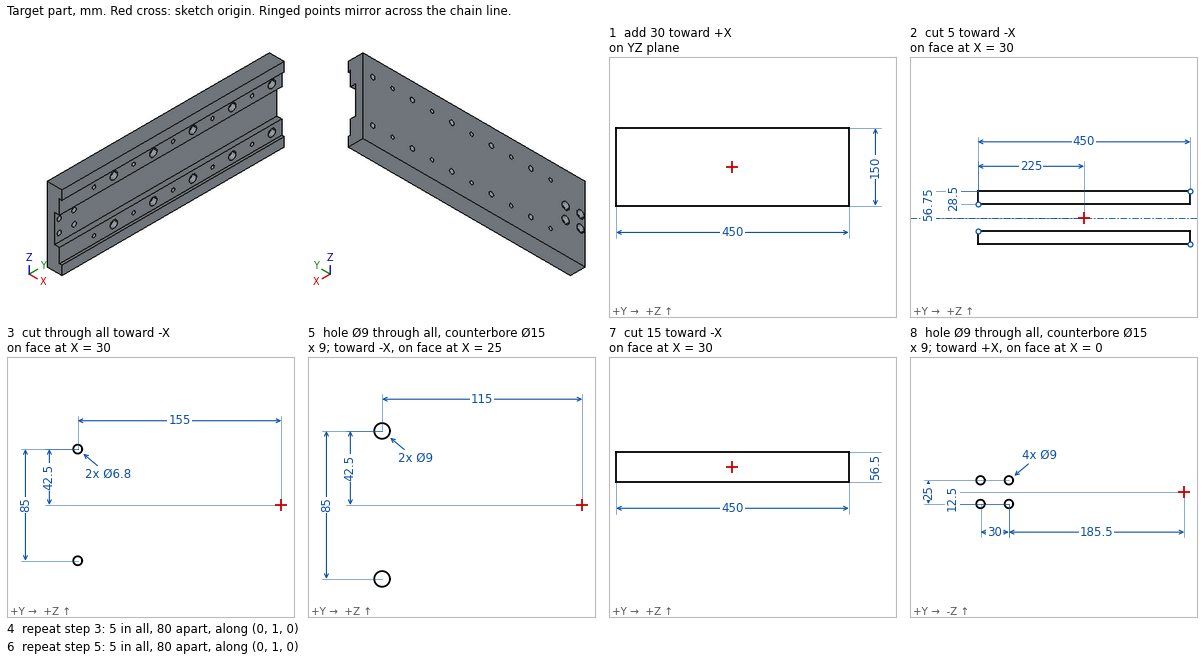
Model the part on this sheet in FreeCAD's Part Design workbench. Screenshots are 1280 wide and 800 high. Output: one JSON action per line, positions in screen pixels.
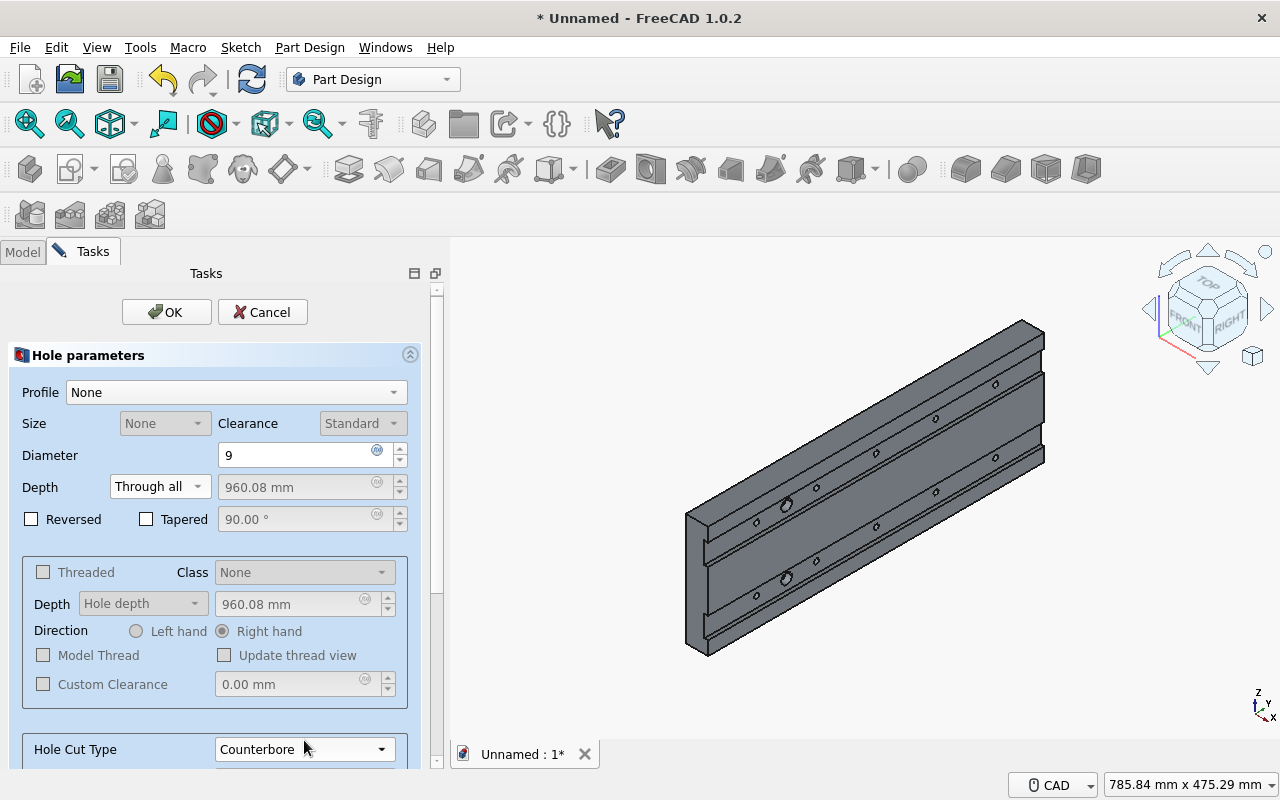
{"action": "scroll", "coordinate": [437, 526], "scroll_direction": "down", "scroll_amount": 2}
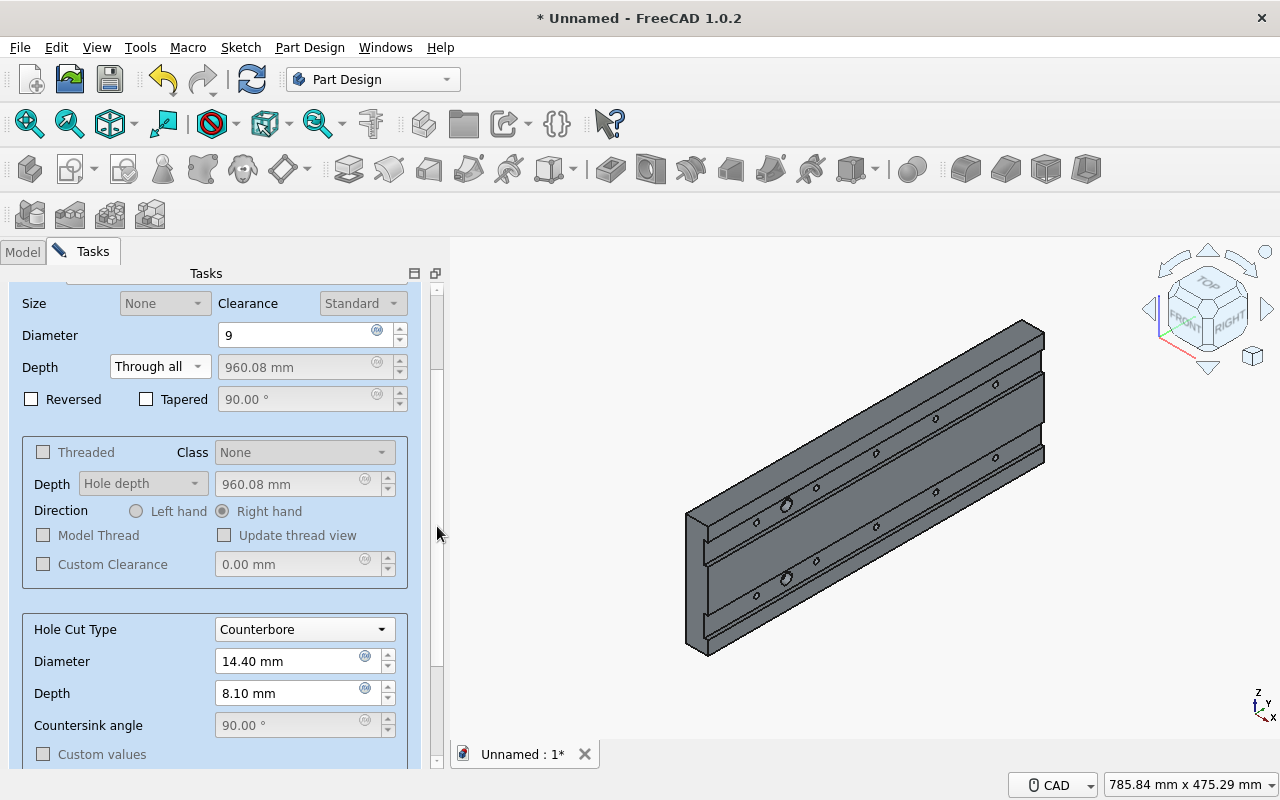
{"action": "triple_click", "coordinate": [298, 661]}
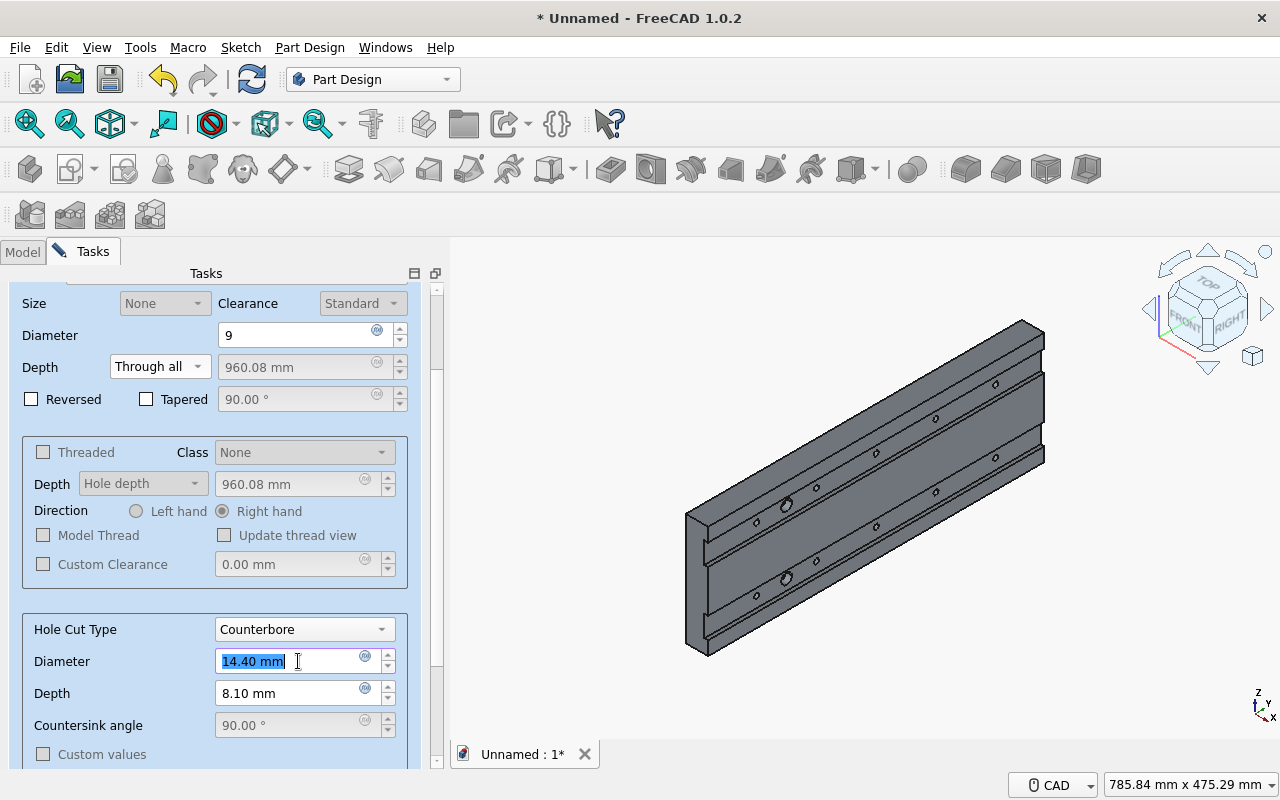
{"action": "type", "text": "15"}
{"action": "key", "text": "Tab"}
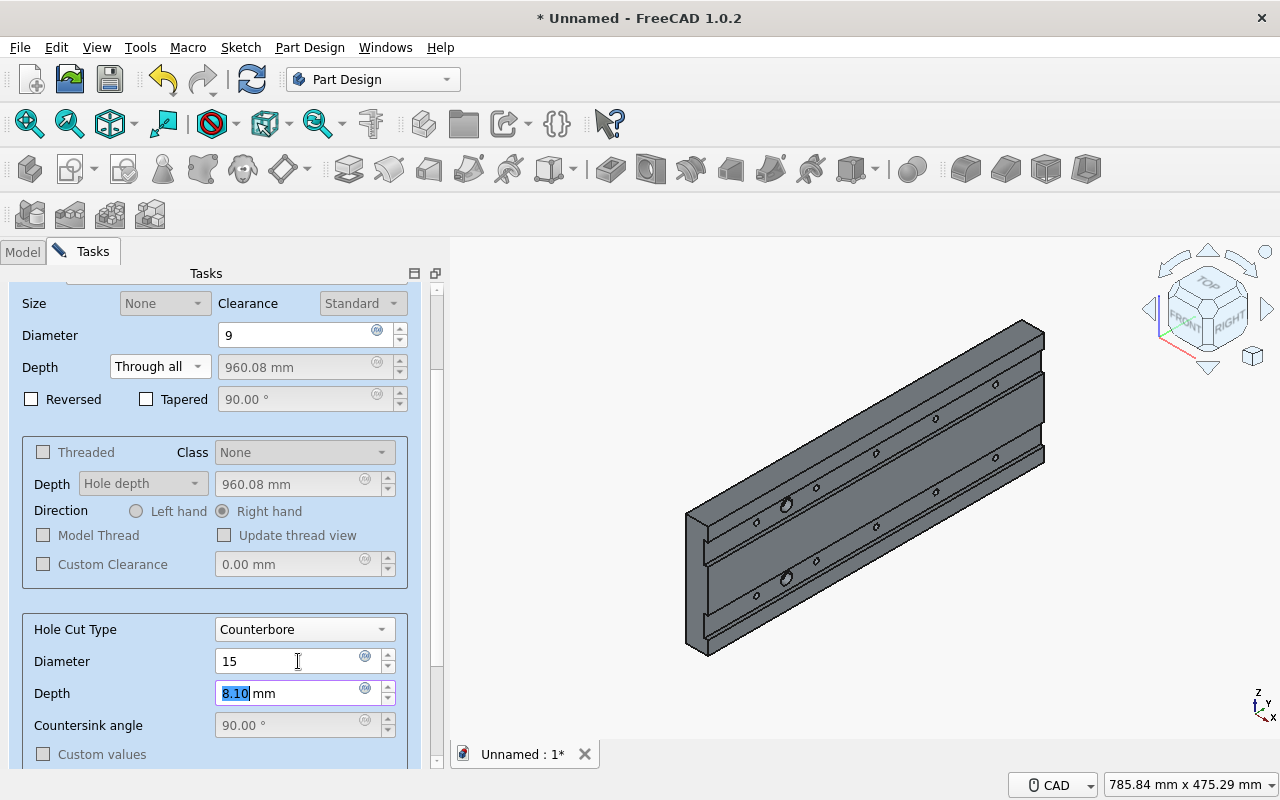
{"action": "type", "text": "9"}
{"action": "key", "text": "Tab"}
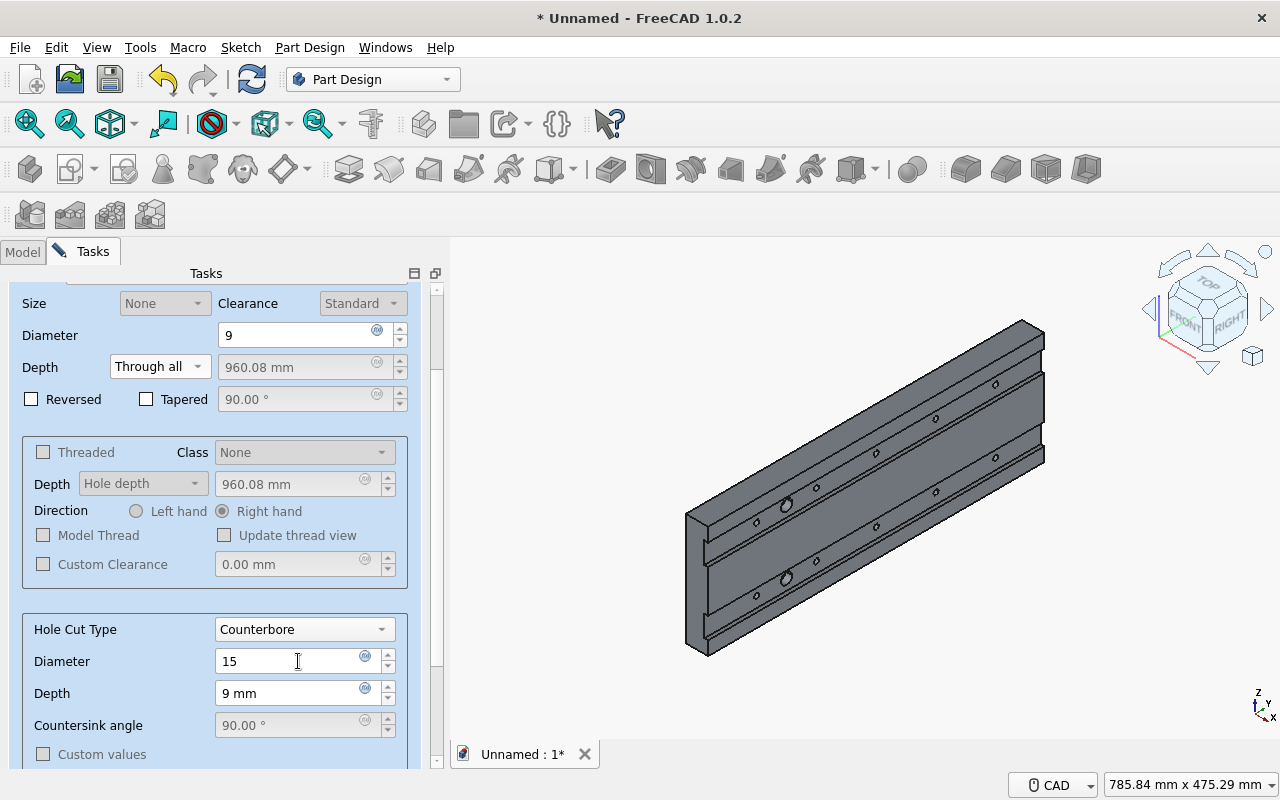
{"action": "scroll", "coordinate": [437, 526], "scroll_direction": "up", "scroll_amount": 3}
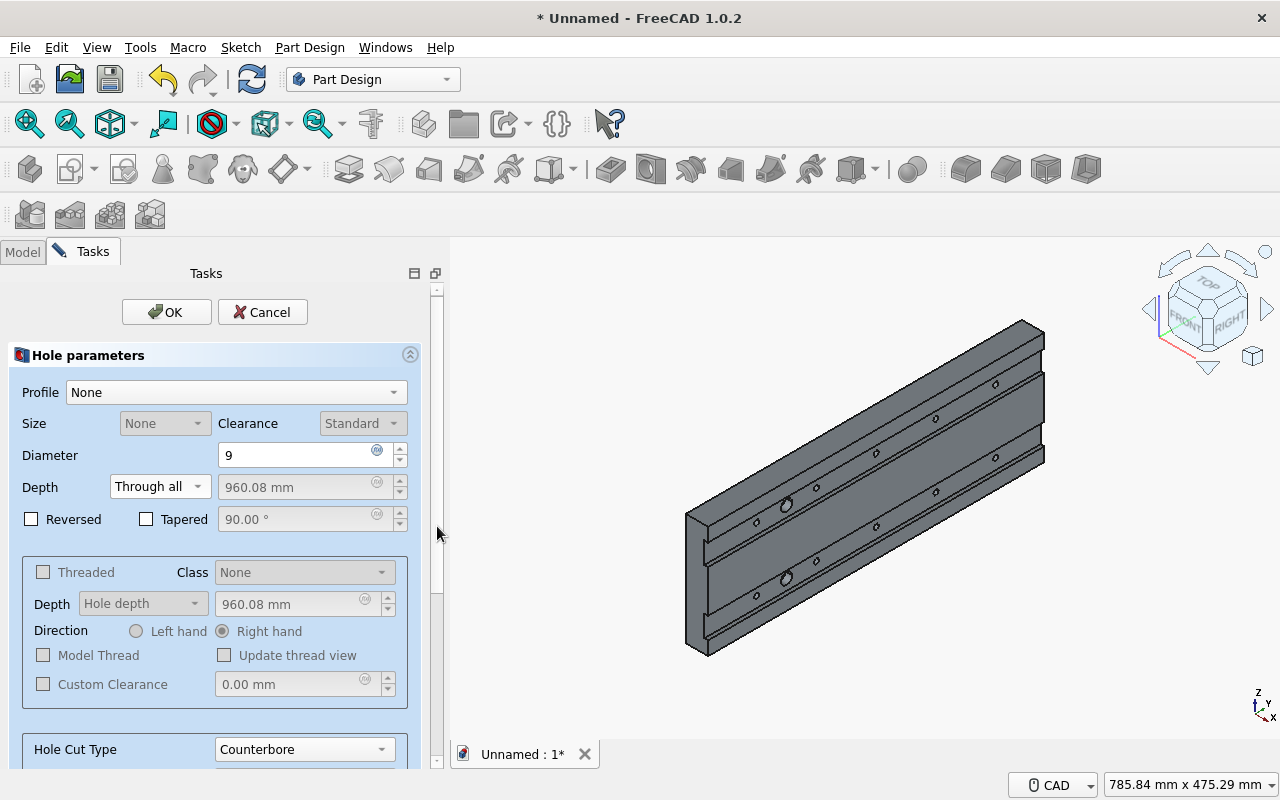
{"action": "left_click", "coordinate": [167, 312]}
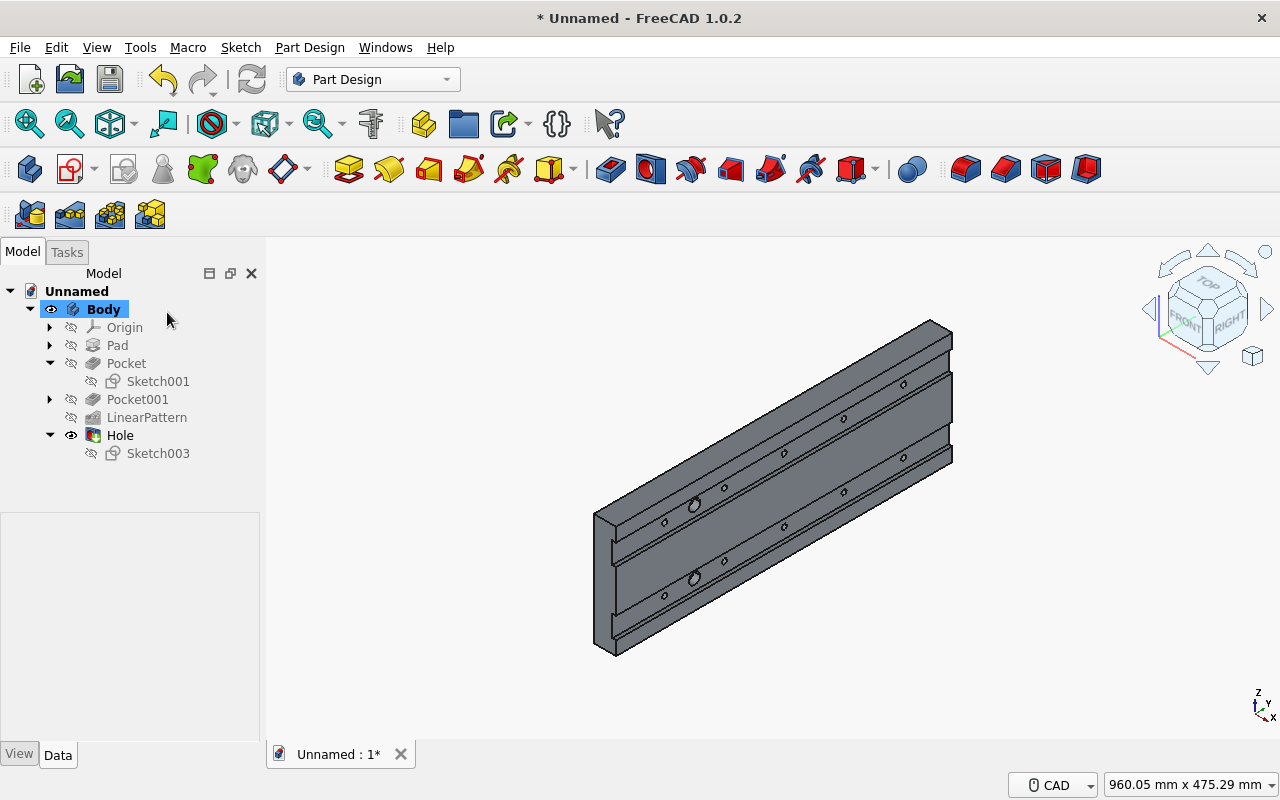
{"action": "left_click", "coordinate": [116, 435]}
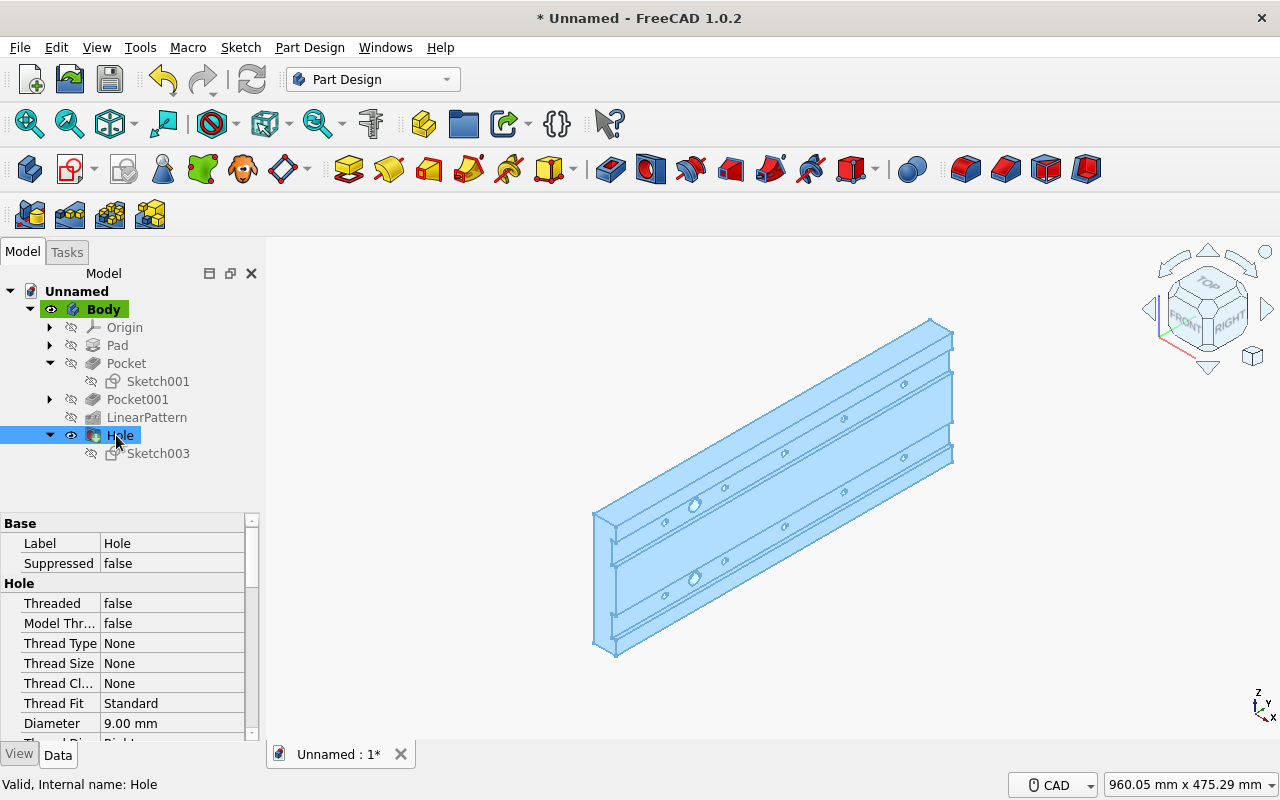
{"action": "left_click", "coordinate": [70, 214]}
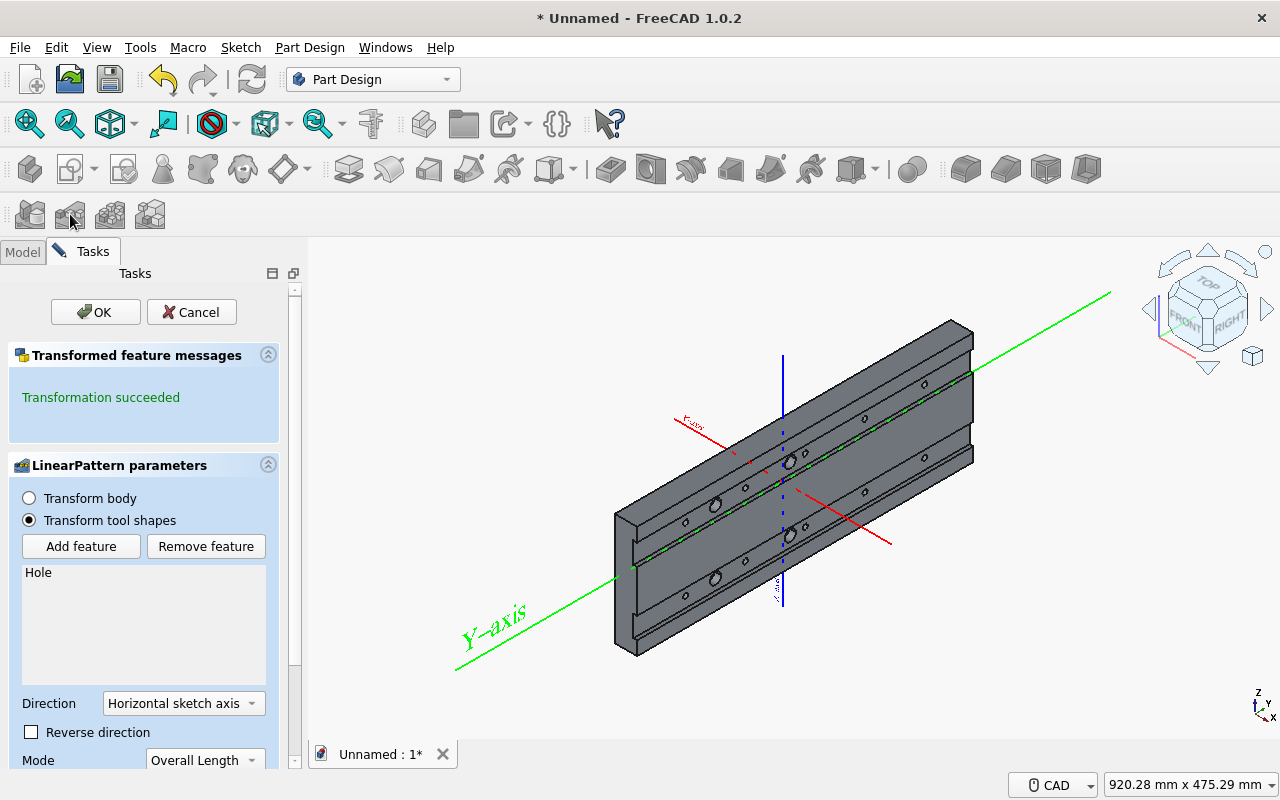
{"action": "left_click", "coordinate": [184, 704]}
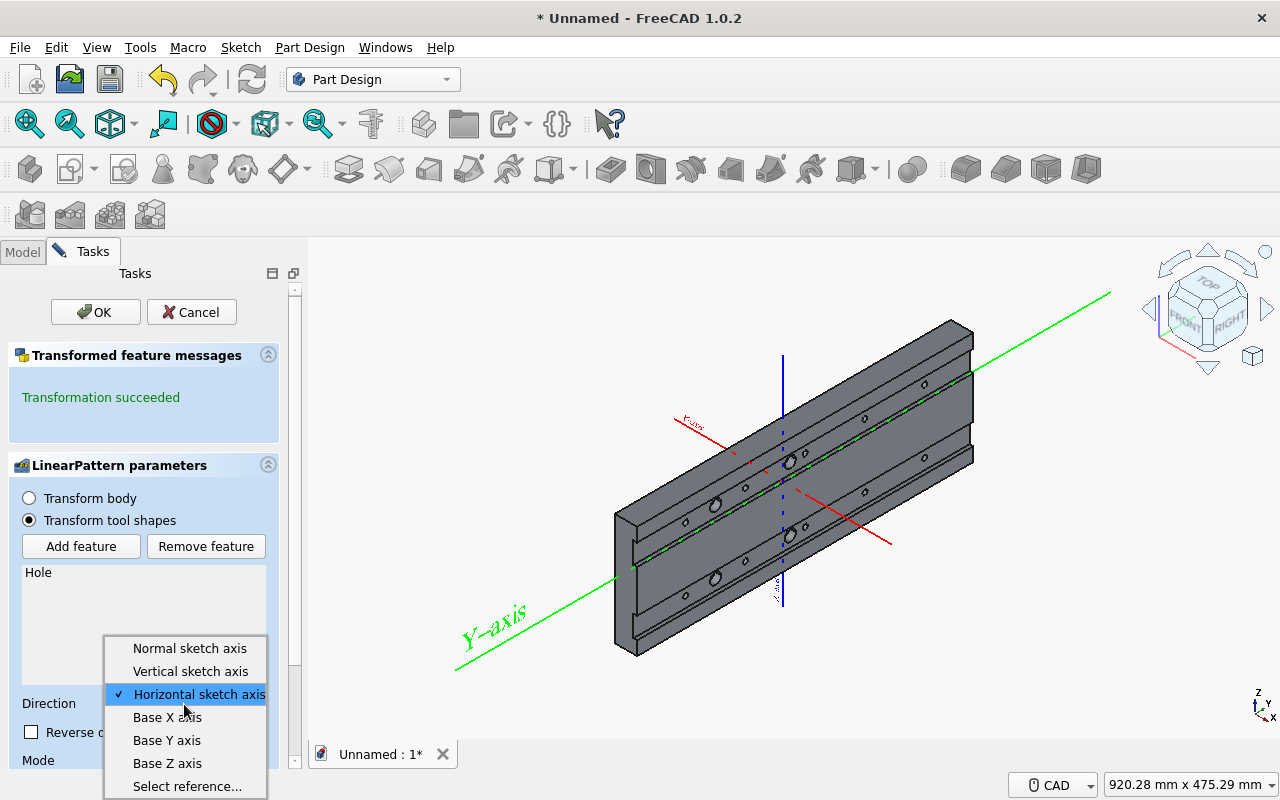
{"action": "left_click", "coordinate": [184, 740]}